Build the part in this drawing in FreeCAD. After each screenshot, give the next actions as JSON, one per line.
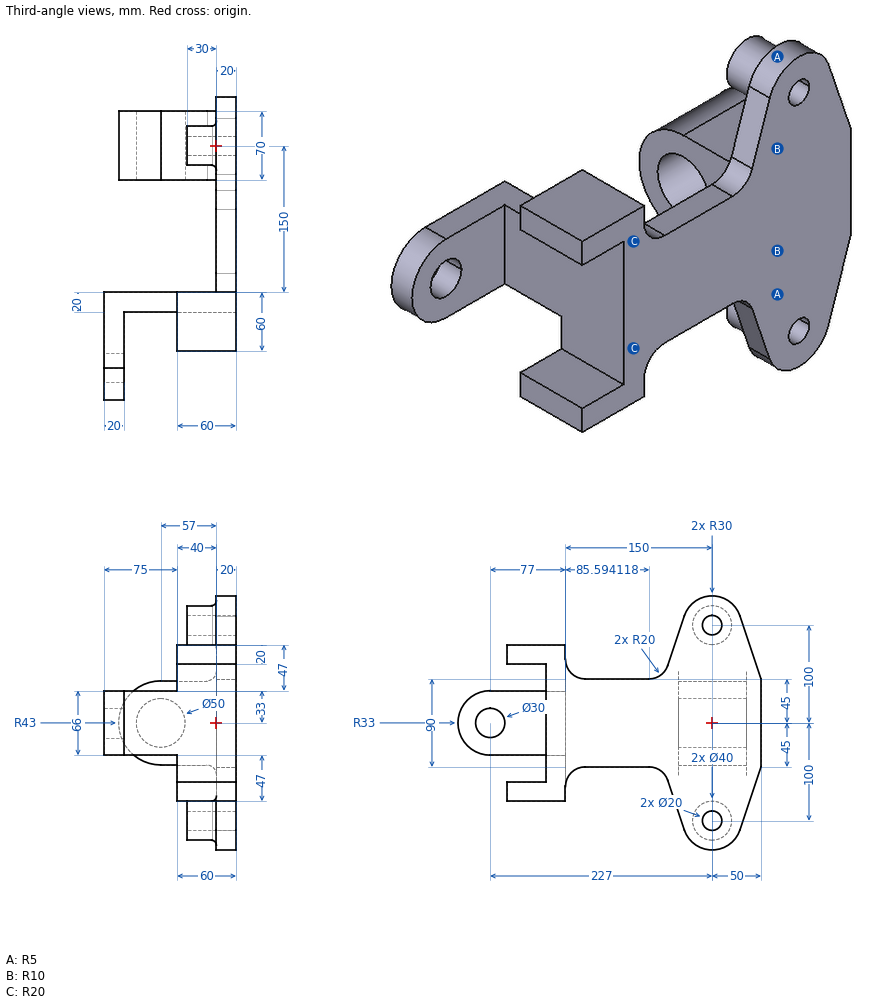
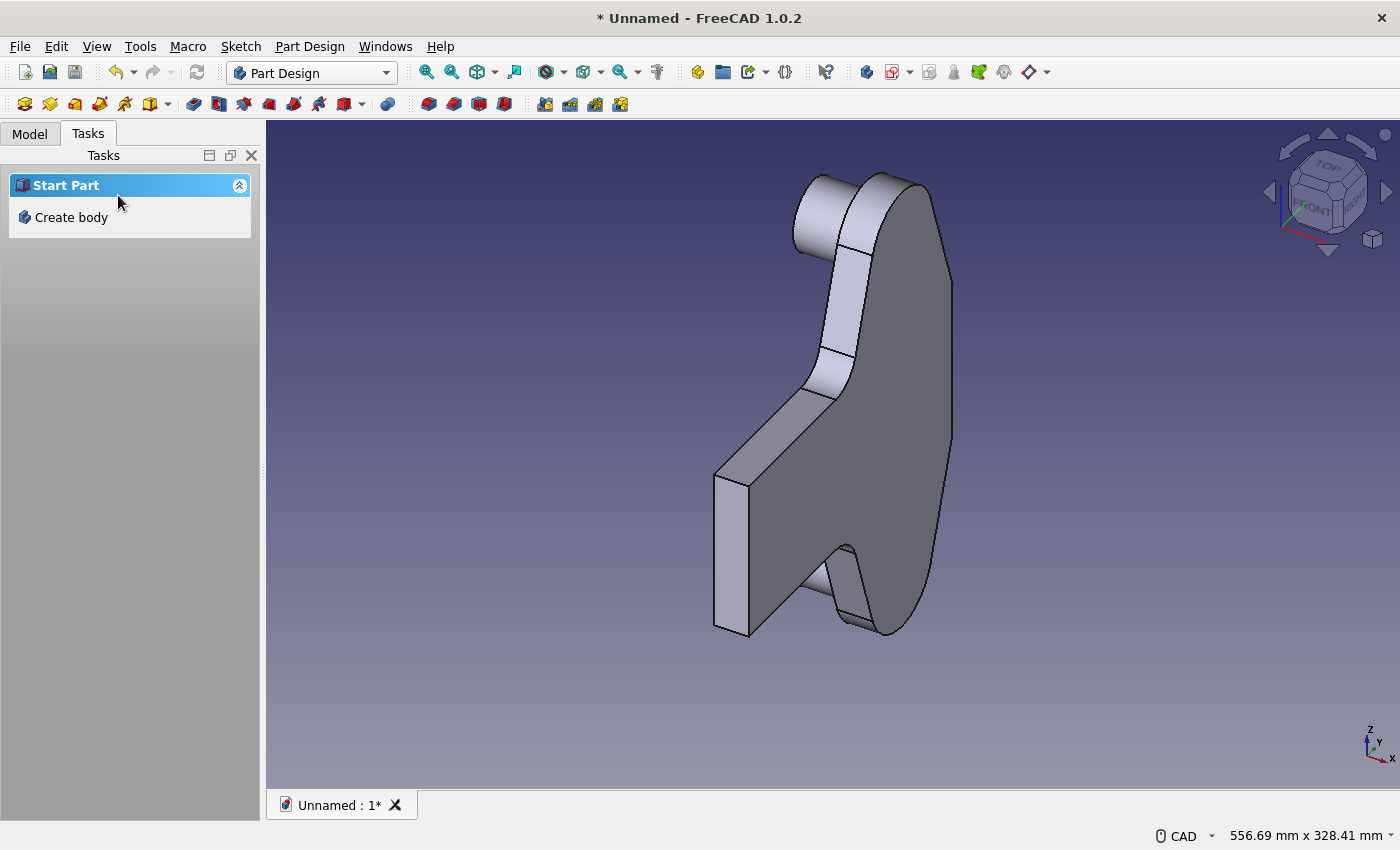
{"action": "left_click", "coordinate": [427, 72]}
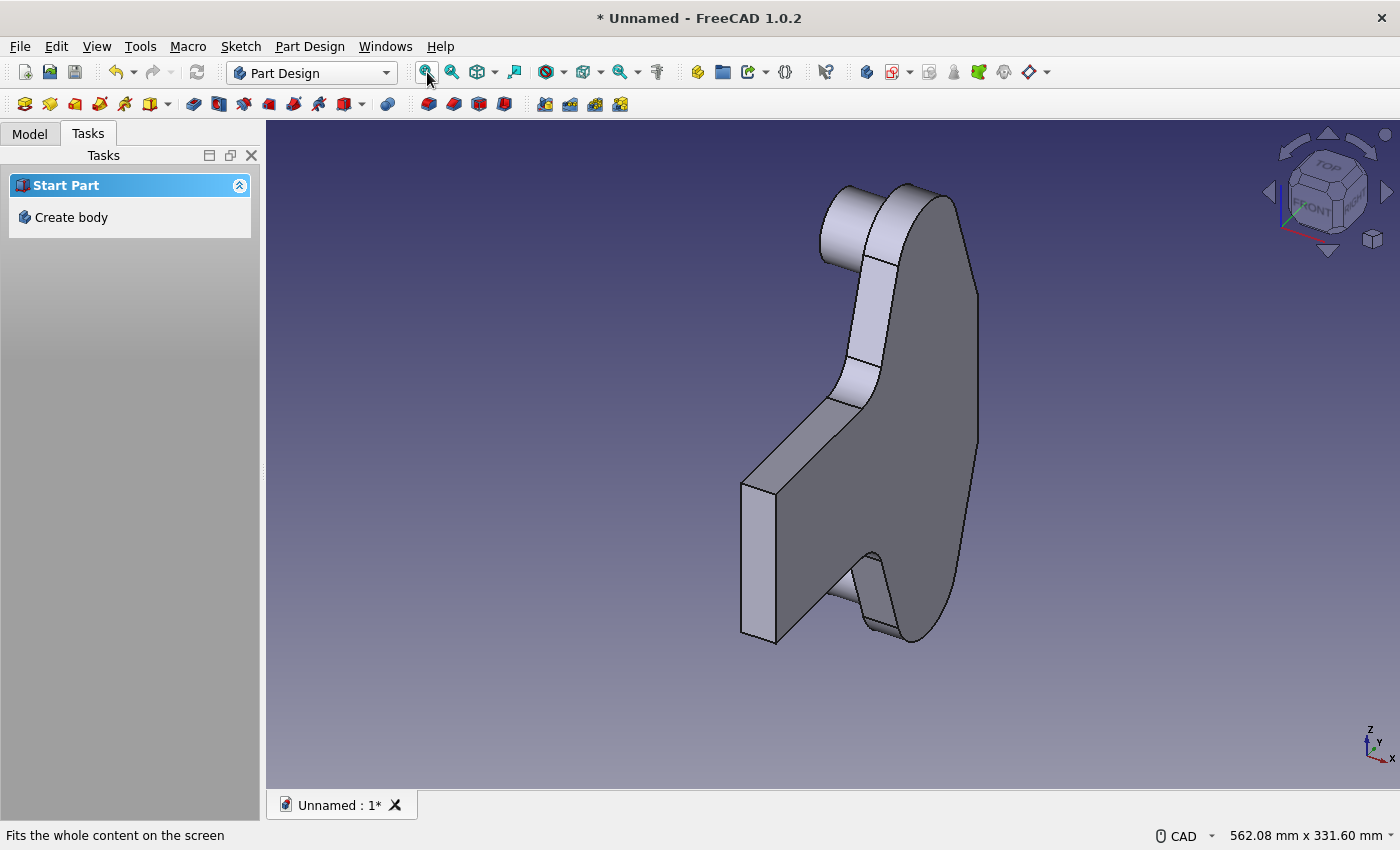
{"action": "key", "text": "6"}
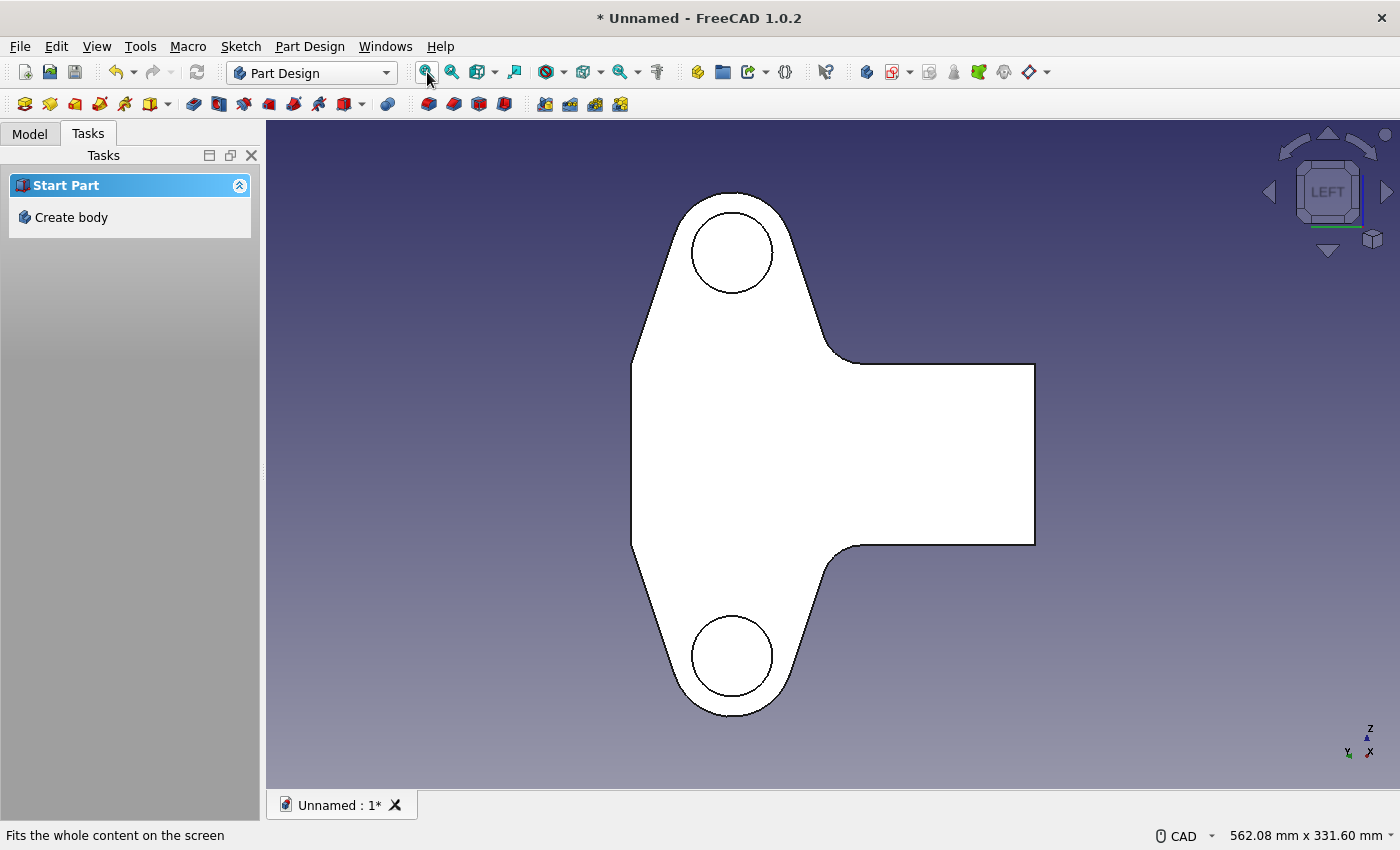
{"action": "left_click", "coordinate": [732, 252]}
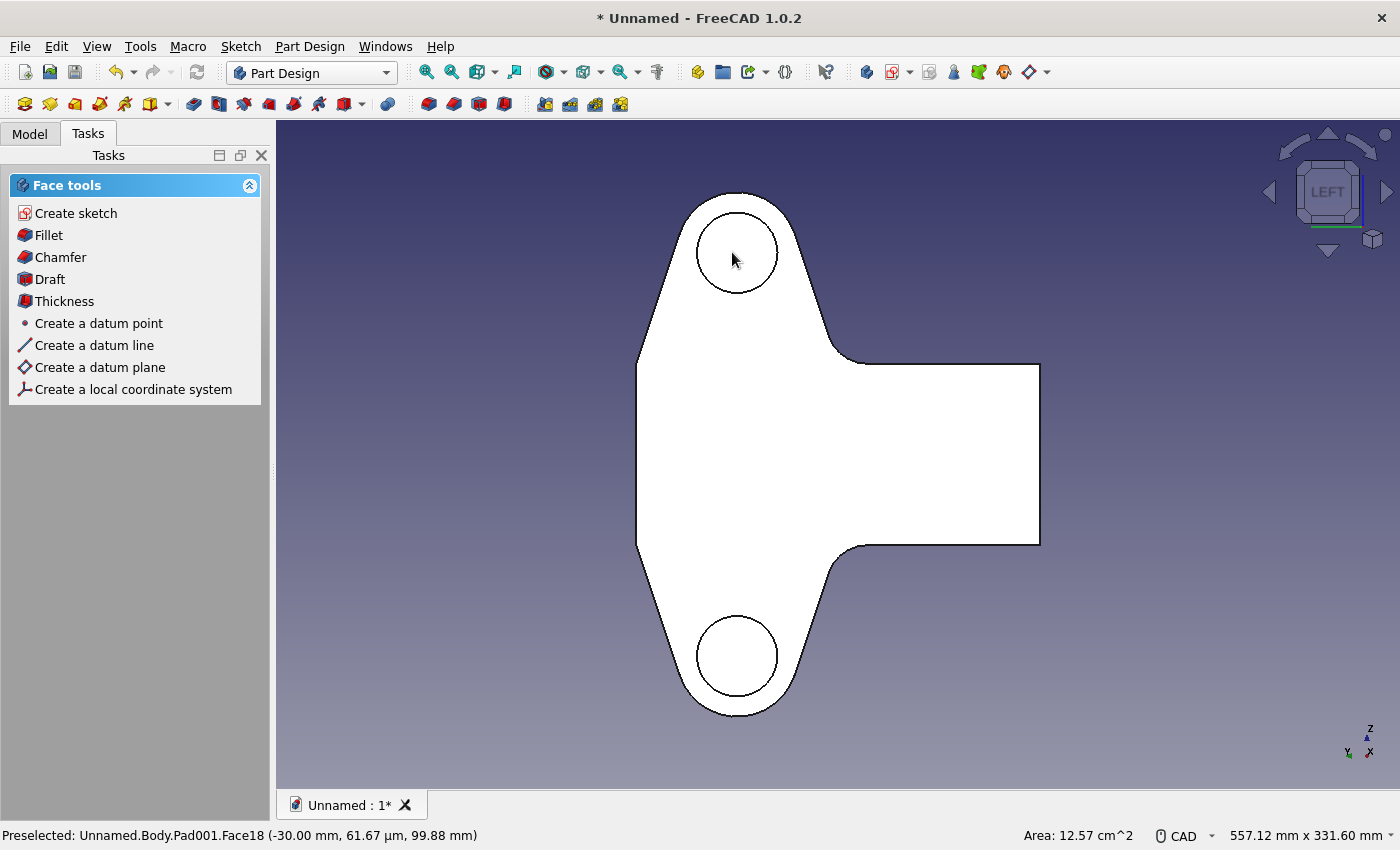
{"action": "left_click", "coordinate": [892, 72]}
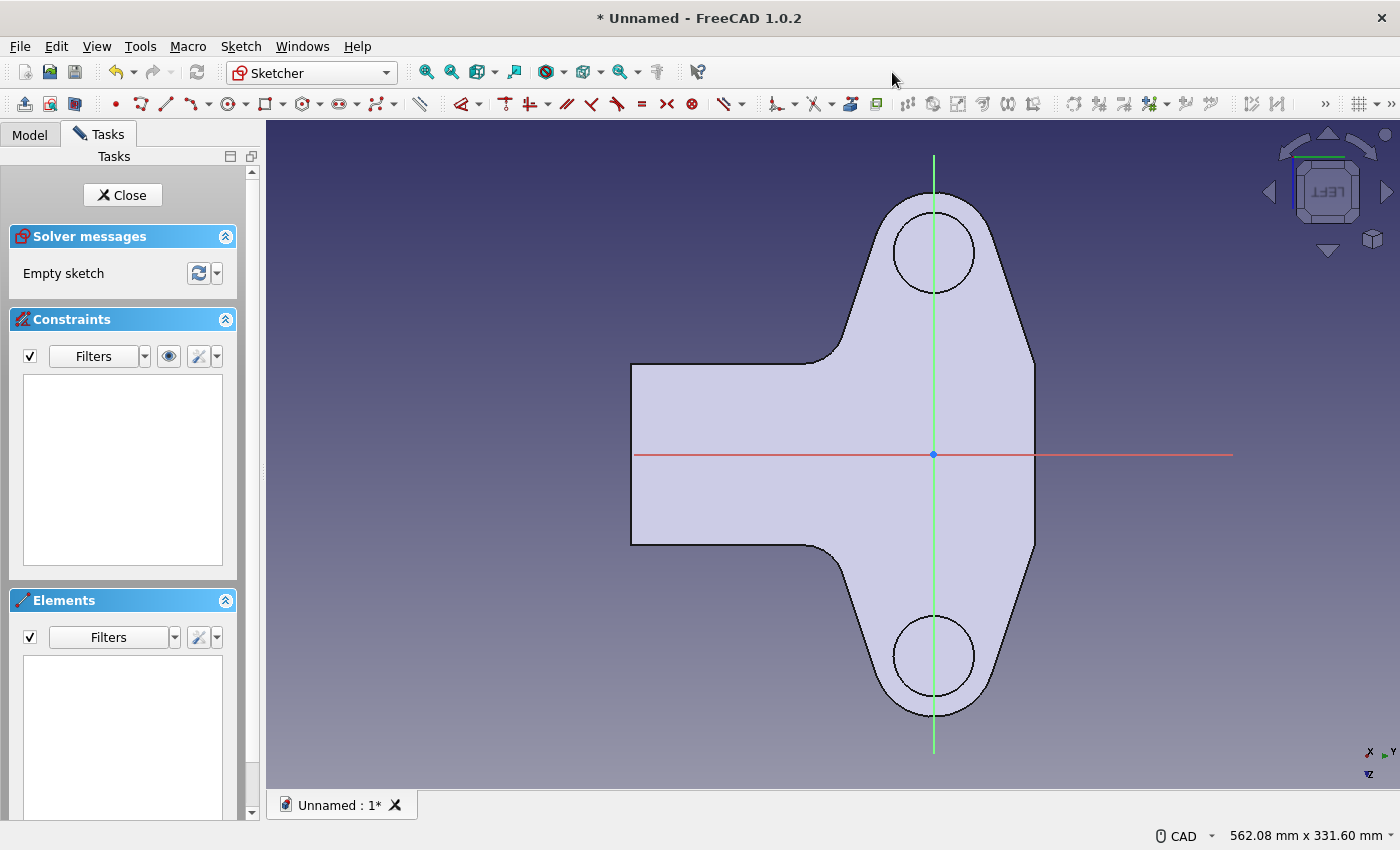
{"action": "key", "text": "g c"}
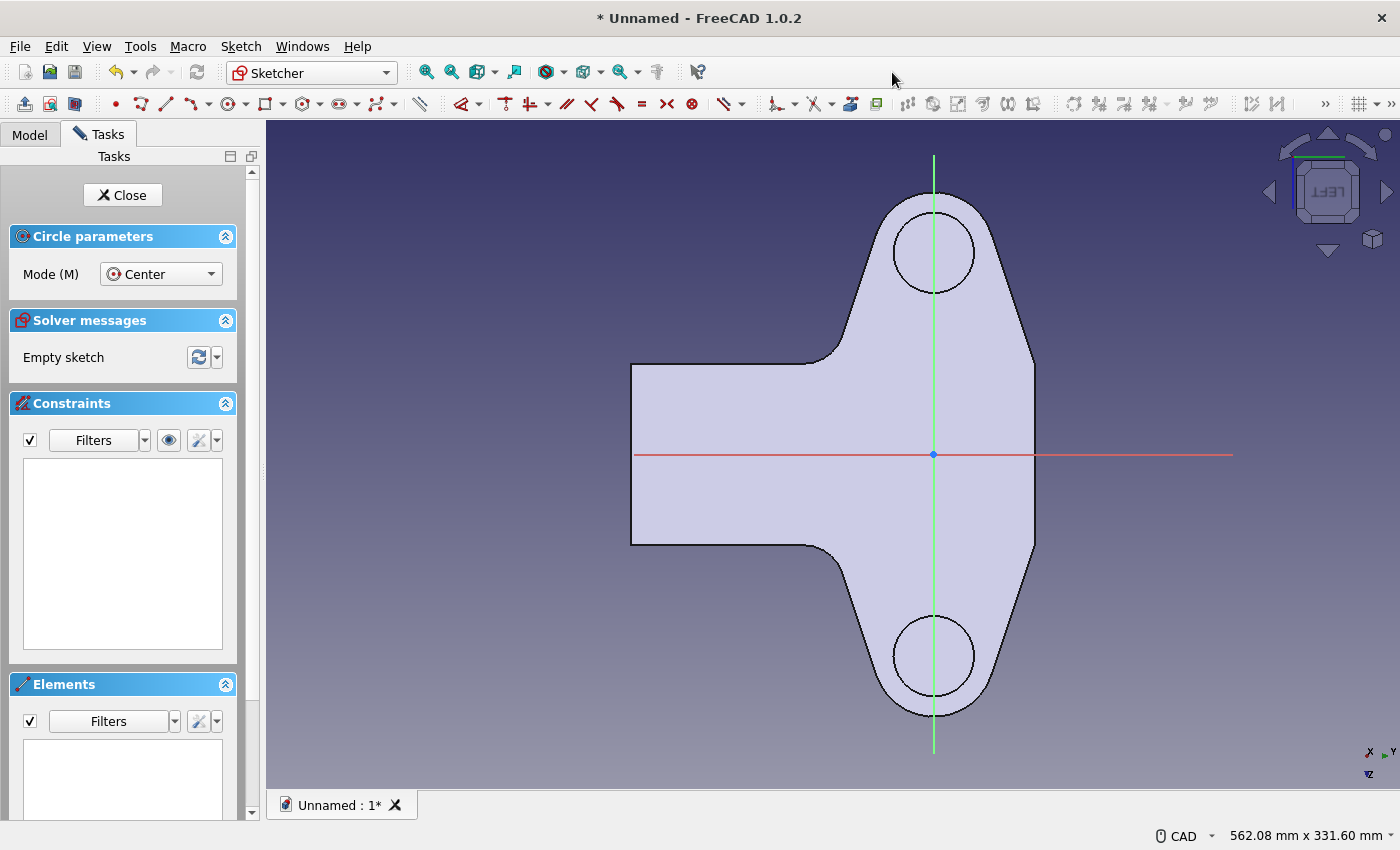
{"action": "left_click", "coordinate": [934, 253]}
{"action": "left_click", "coordinate": [948, 238]}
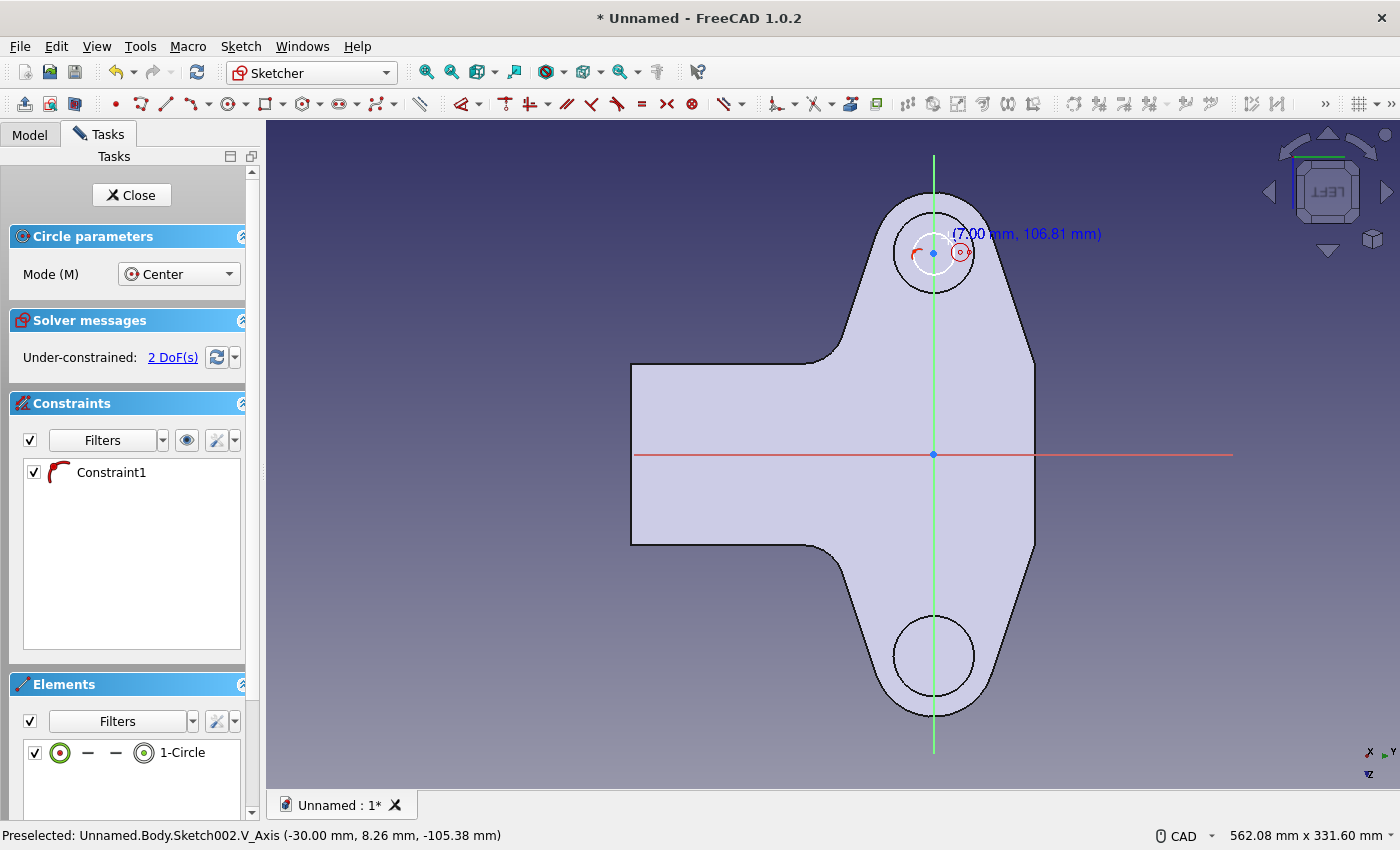
{"action": "left_click", "coordinate": [934, 656]}
{"action": "left_click", "coordinate": [948, 642]}
{"action": "key", "text": "Escape"}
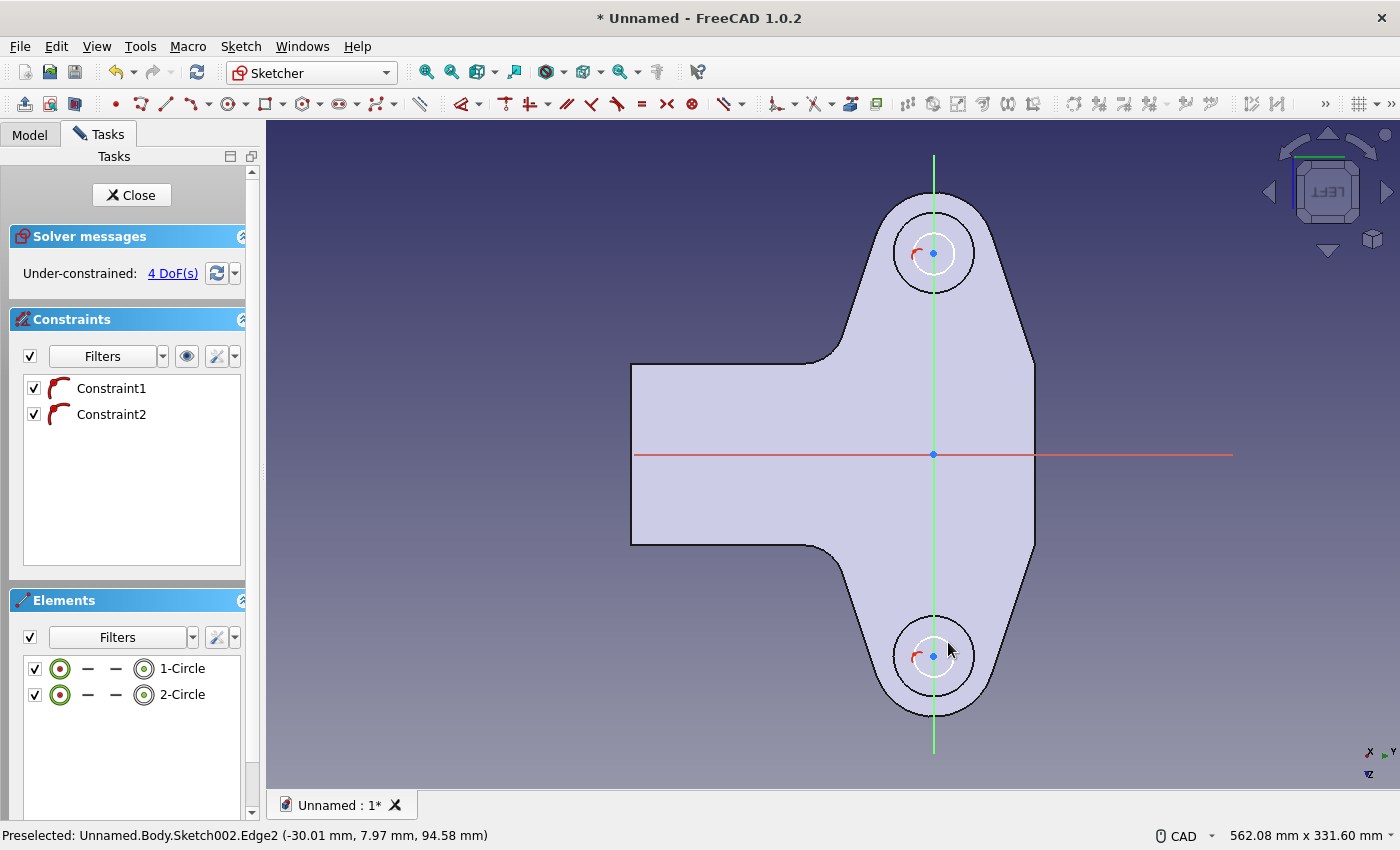
{"action": "left_click", "coordinate": [948, 239]}